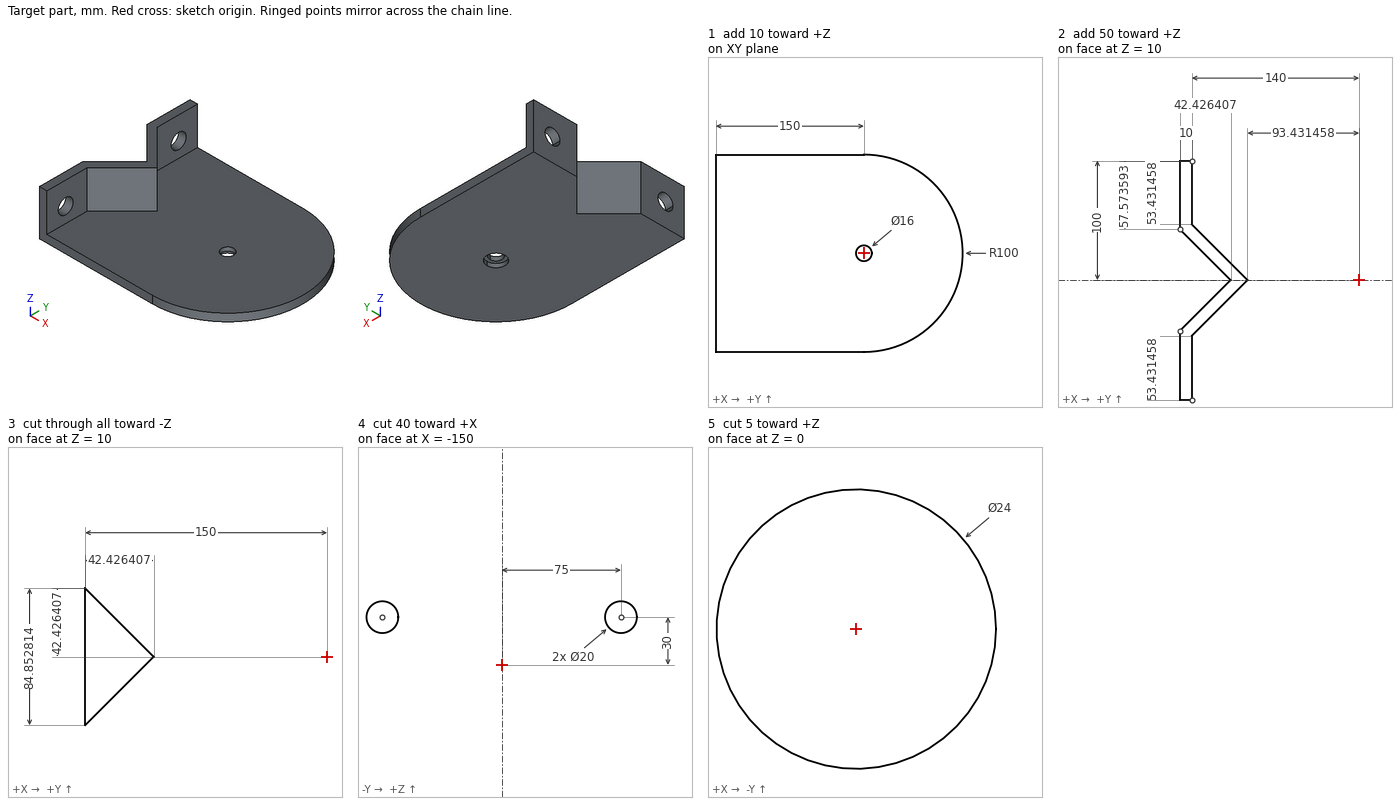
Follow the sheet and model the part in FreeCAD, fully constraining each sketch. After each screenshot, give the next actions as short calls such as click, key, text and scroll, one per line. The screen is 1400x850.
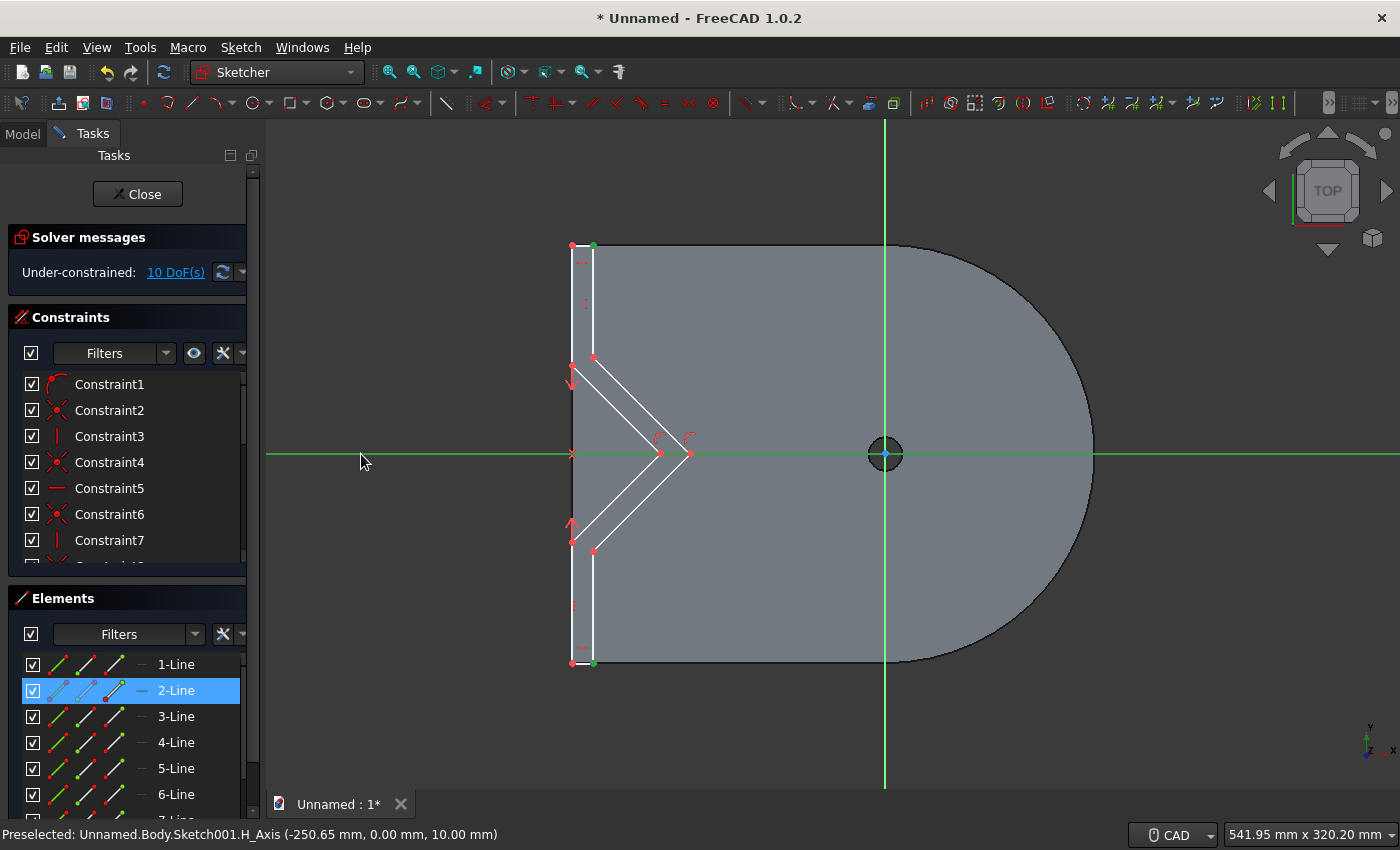
click(690, 104)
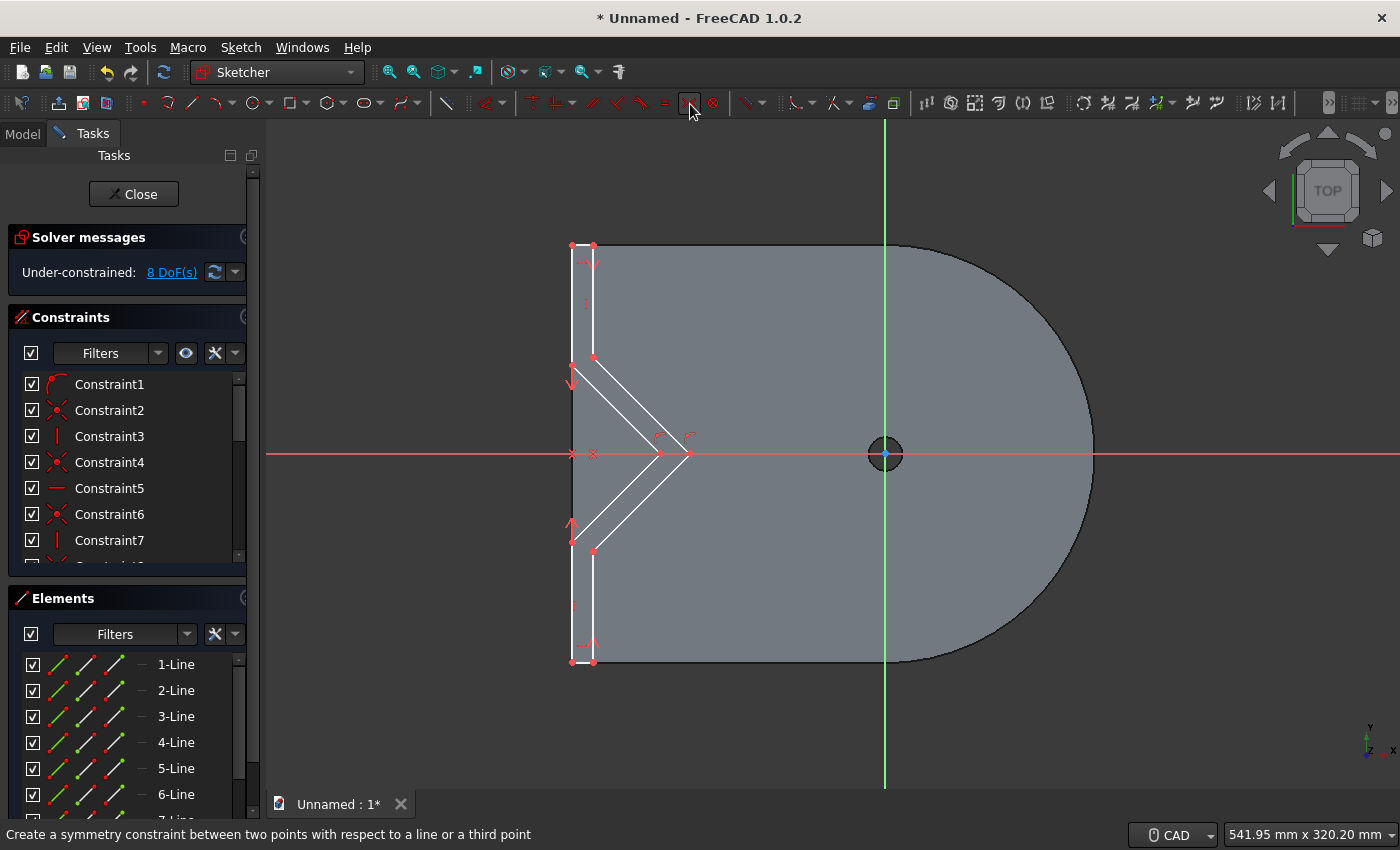
click(486, 104)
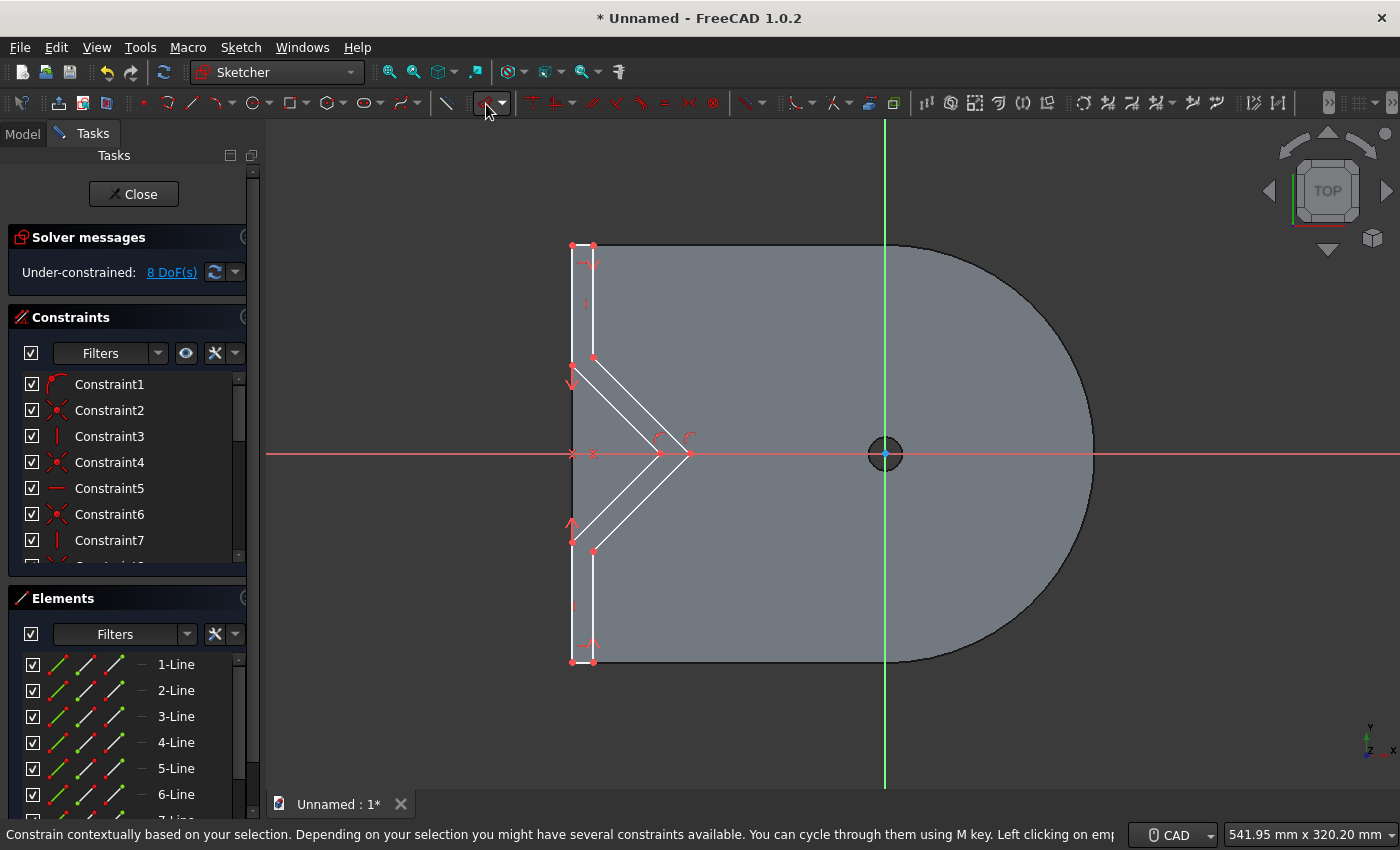
scroll(583, 245, up, 4)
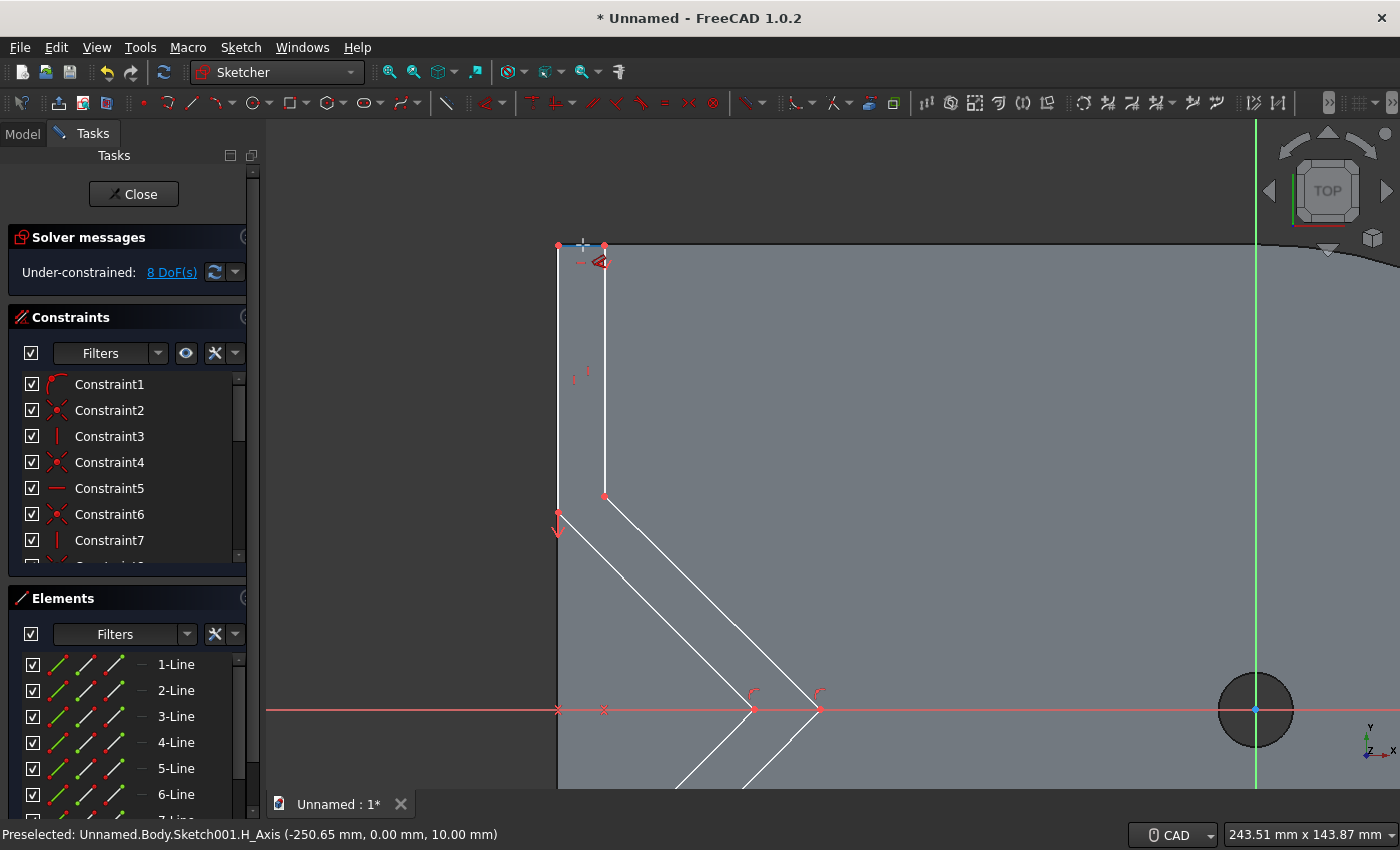
click(582, 246)
click(582, 212)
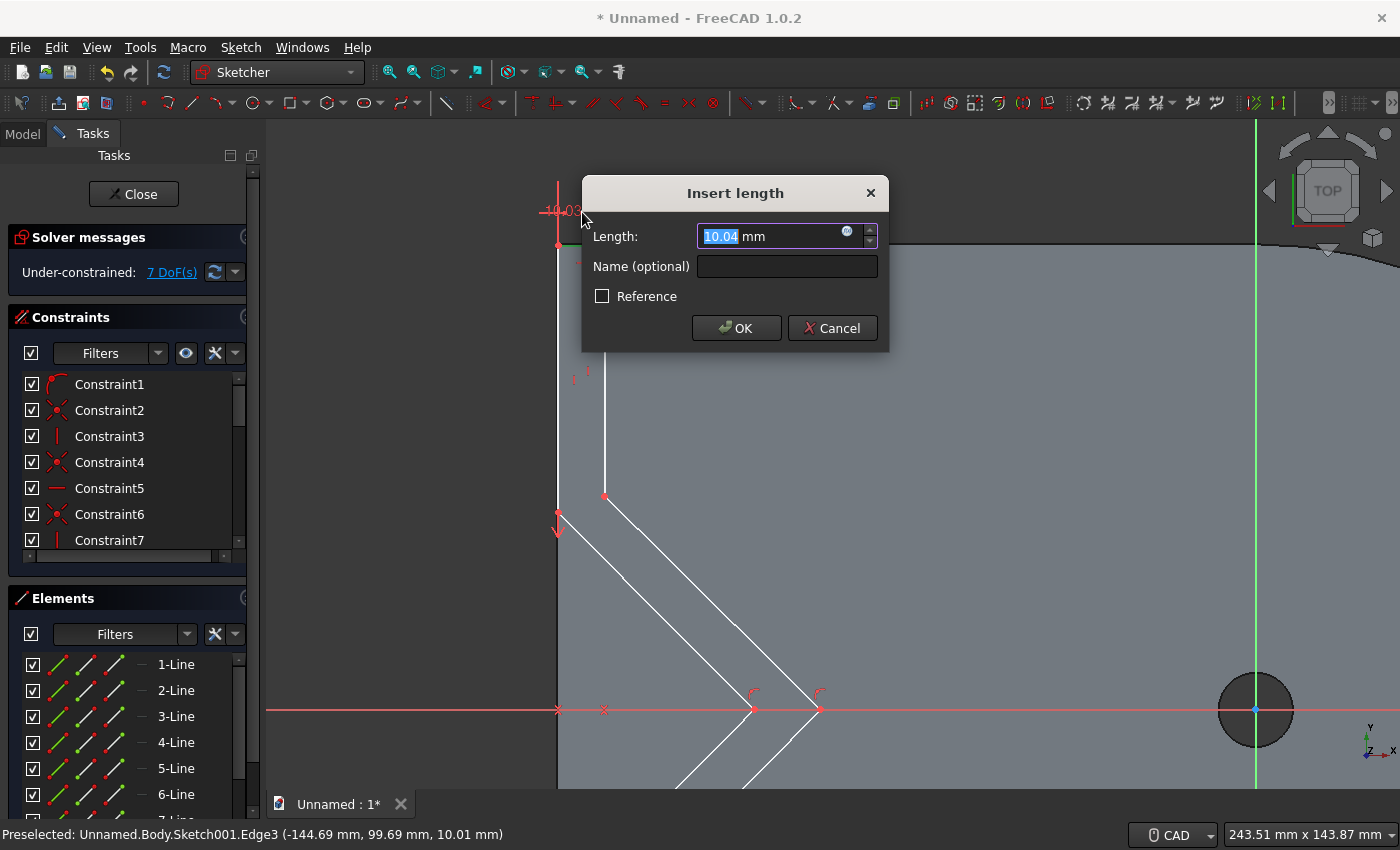
text(10)
key(Return)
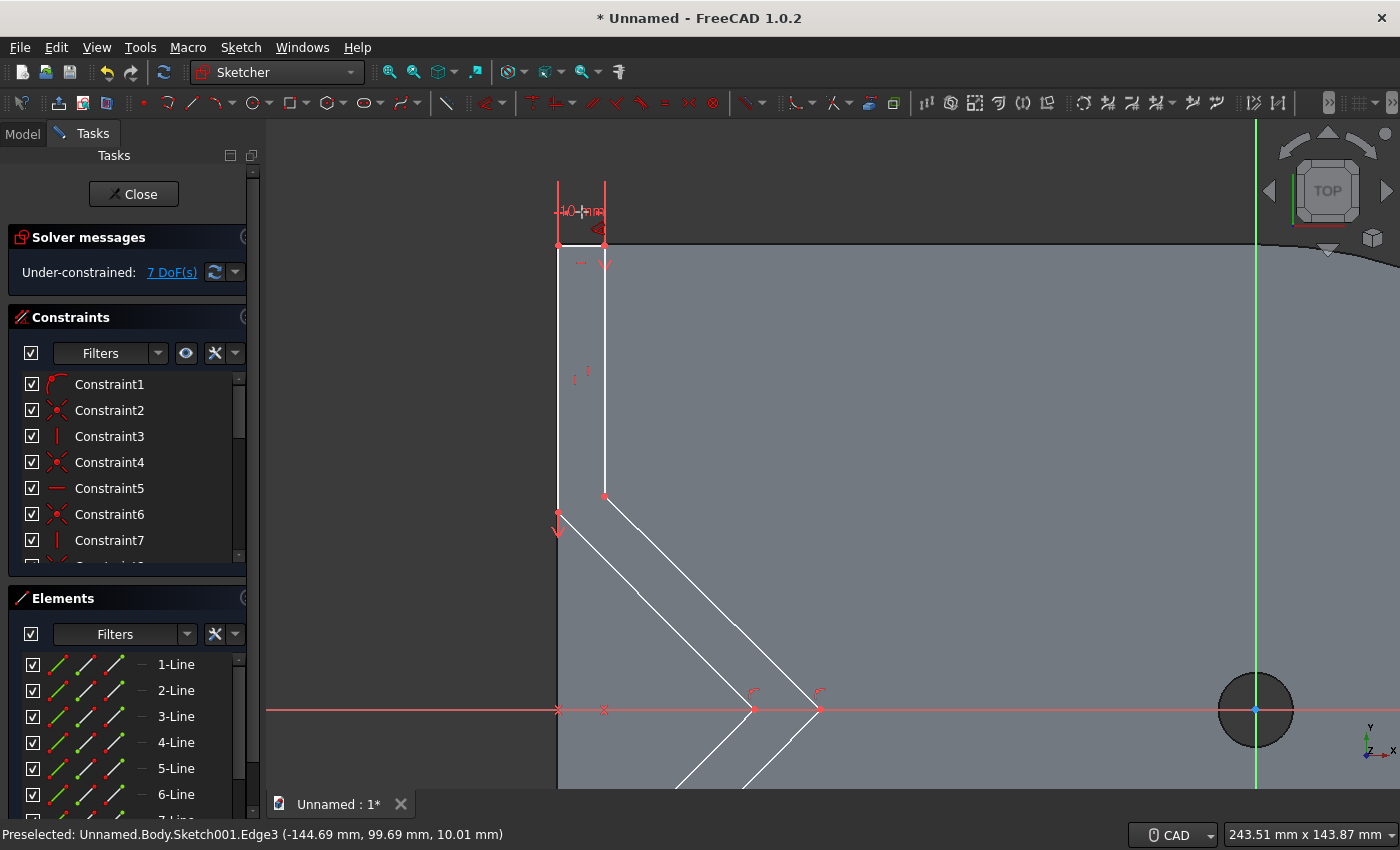
click(605, 496)
click(920, 462)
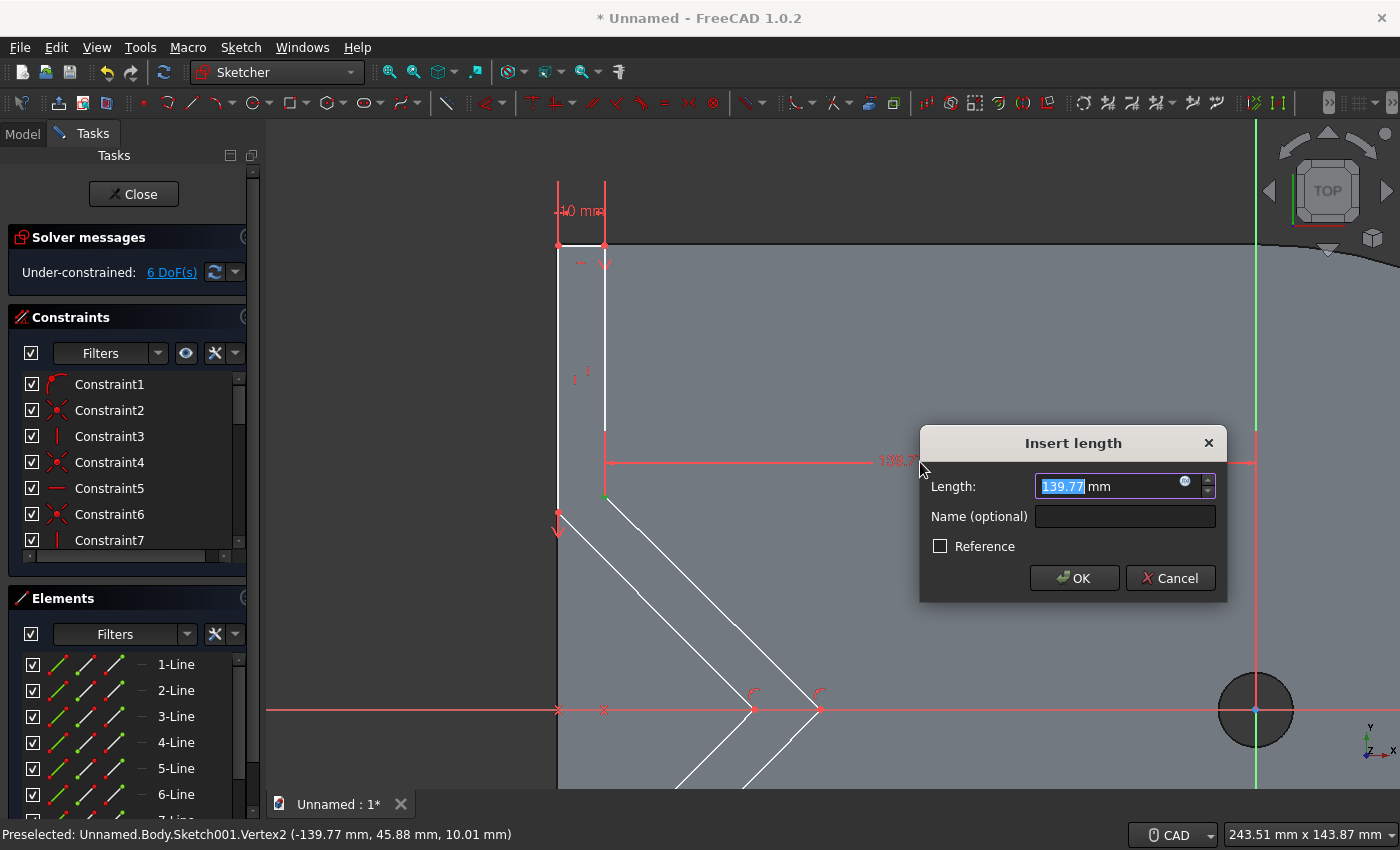
text(140)
key(Return)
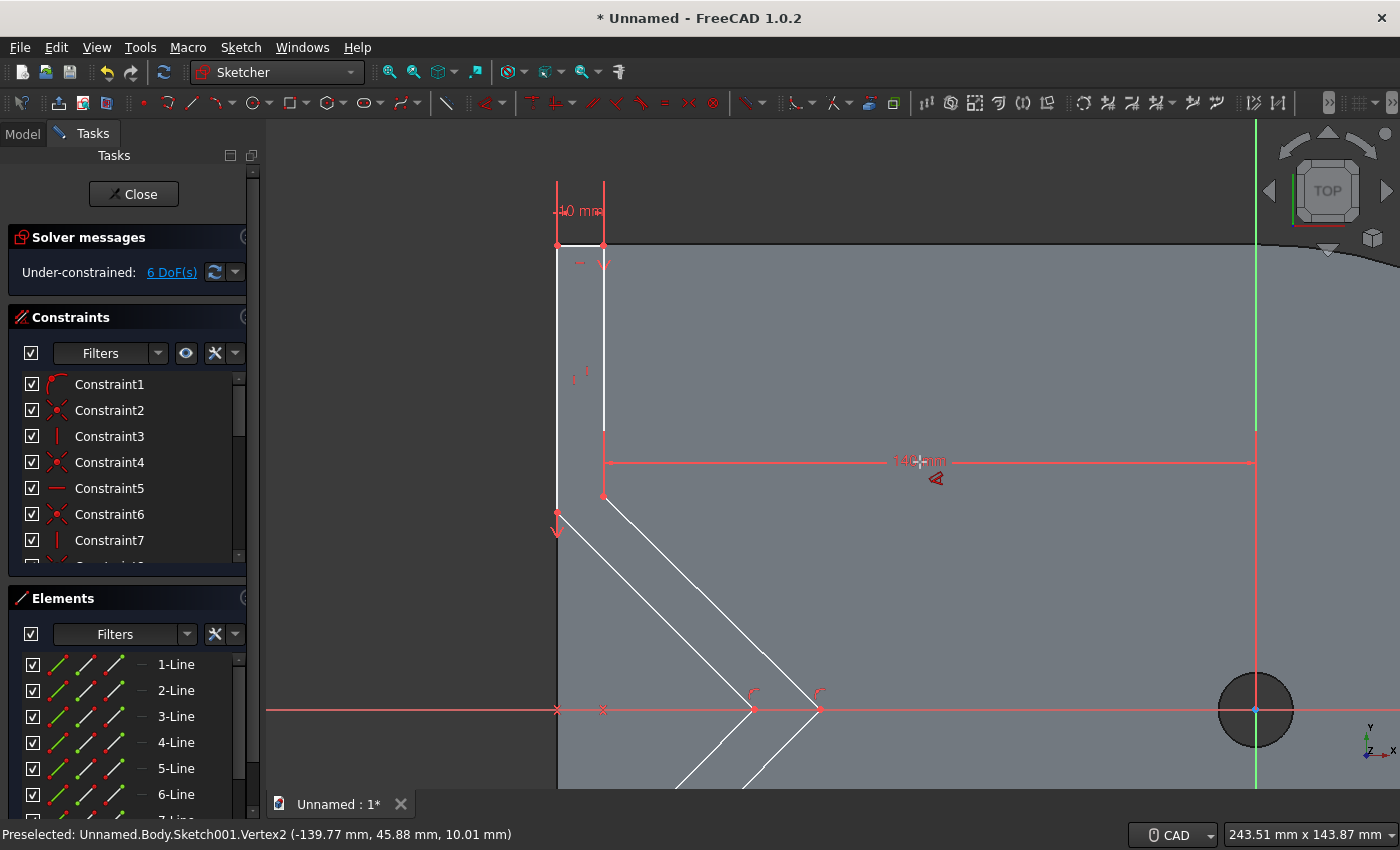
click(604, 246)
click(570, 585)